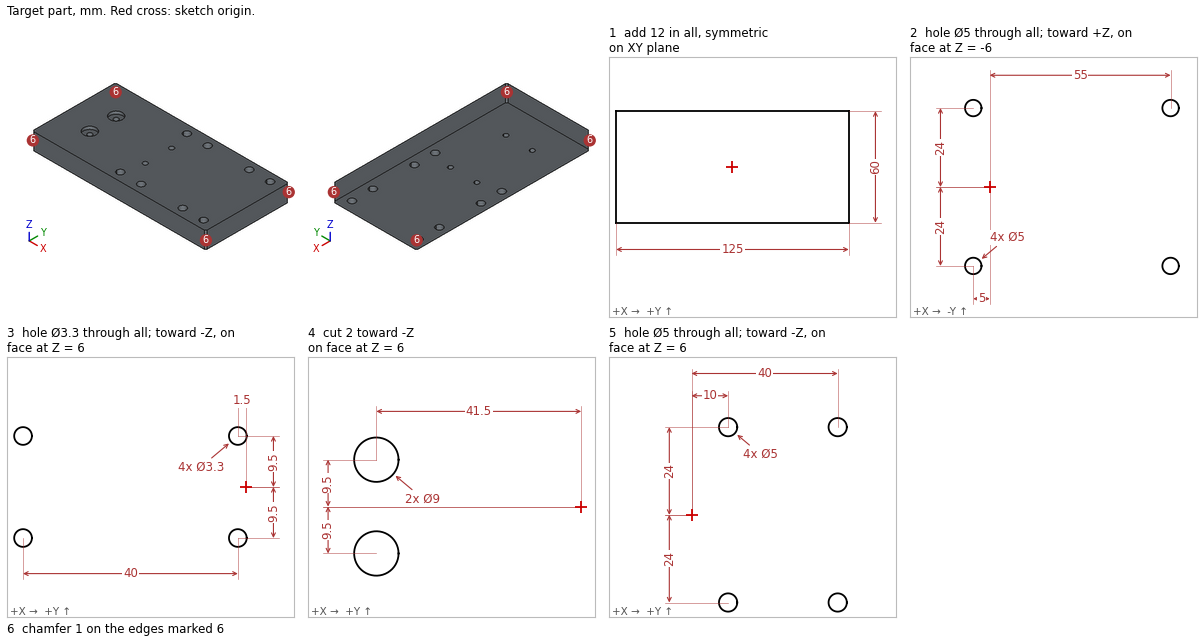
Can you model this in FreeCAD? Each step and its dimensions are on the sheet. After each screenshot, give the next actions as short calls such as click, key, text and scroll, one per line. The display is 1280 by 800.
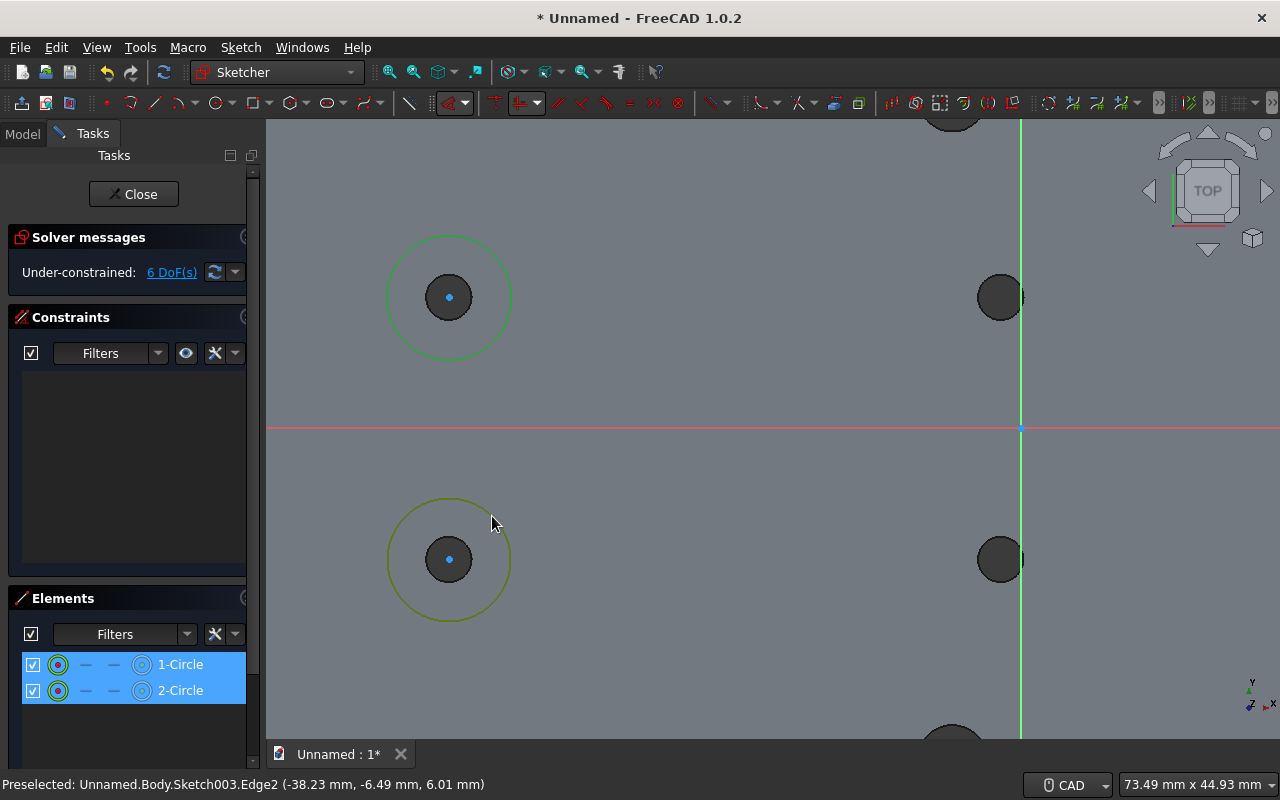
click(630, 104)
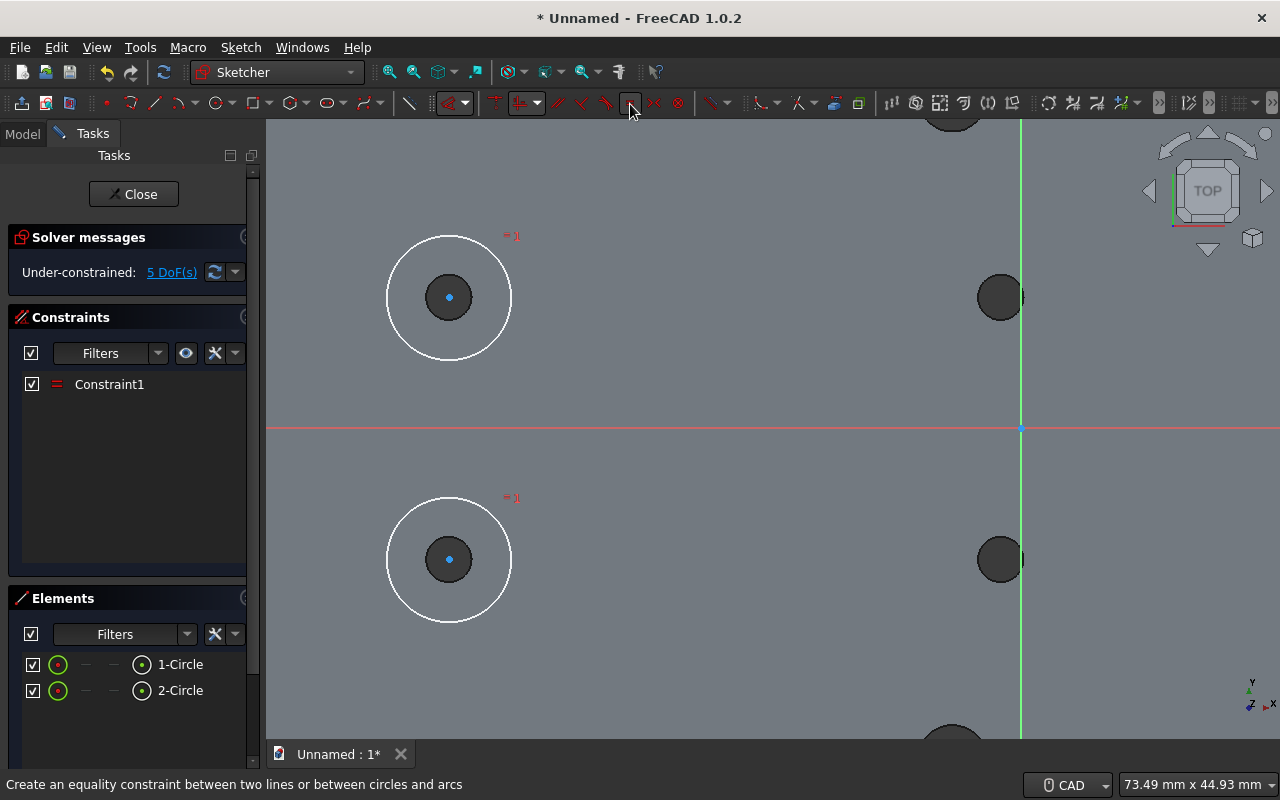
click(449, 298)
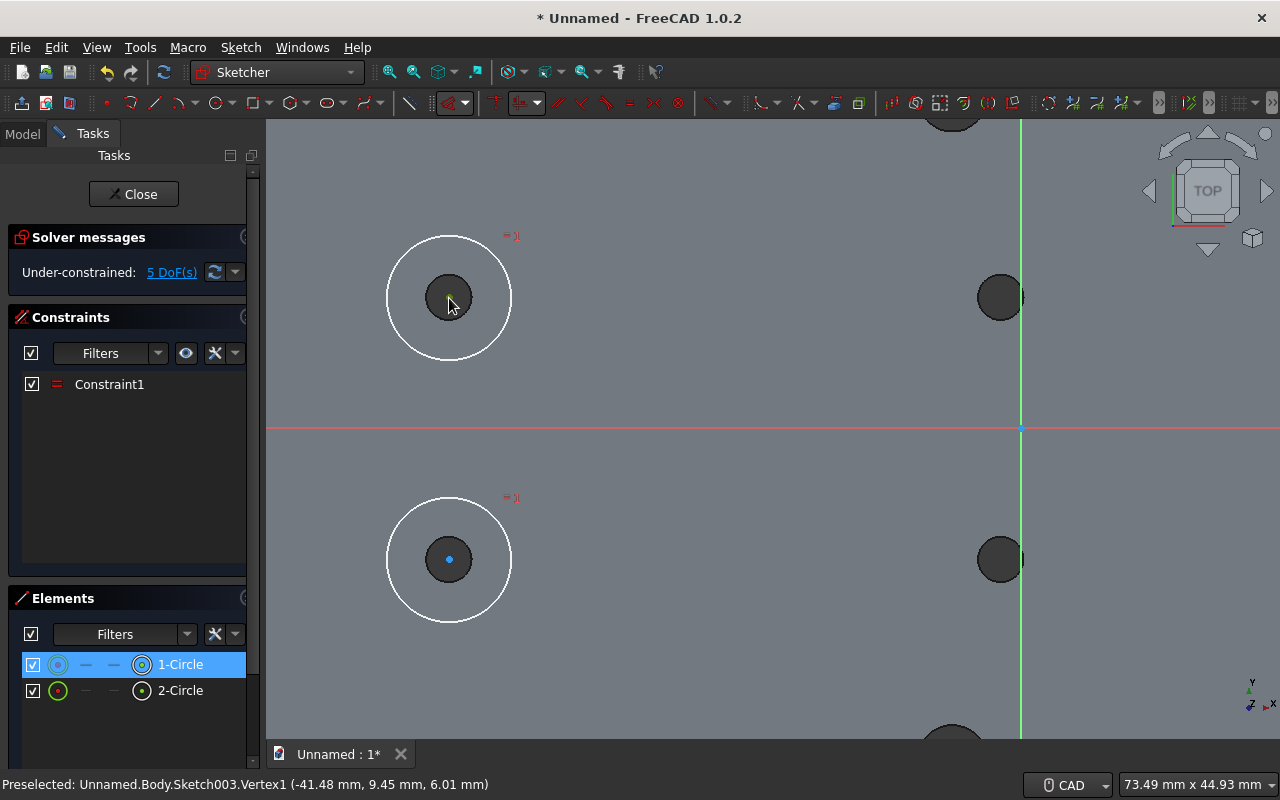
click(449, 560)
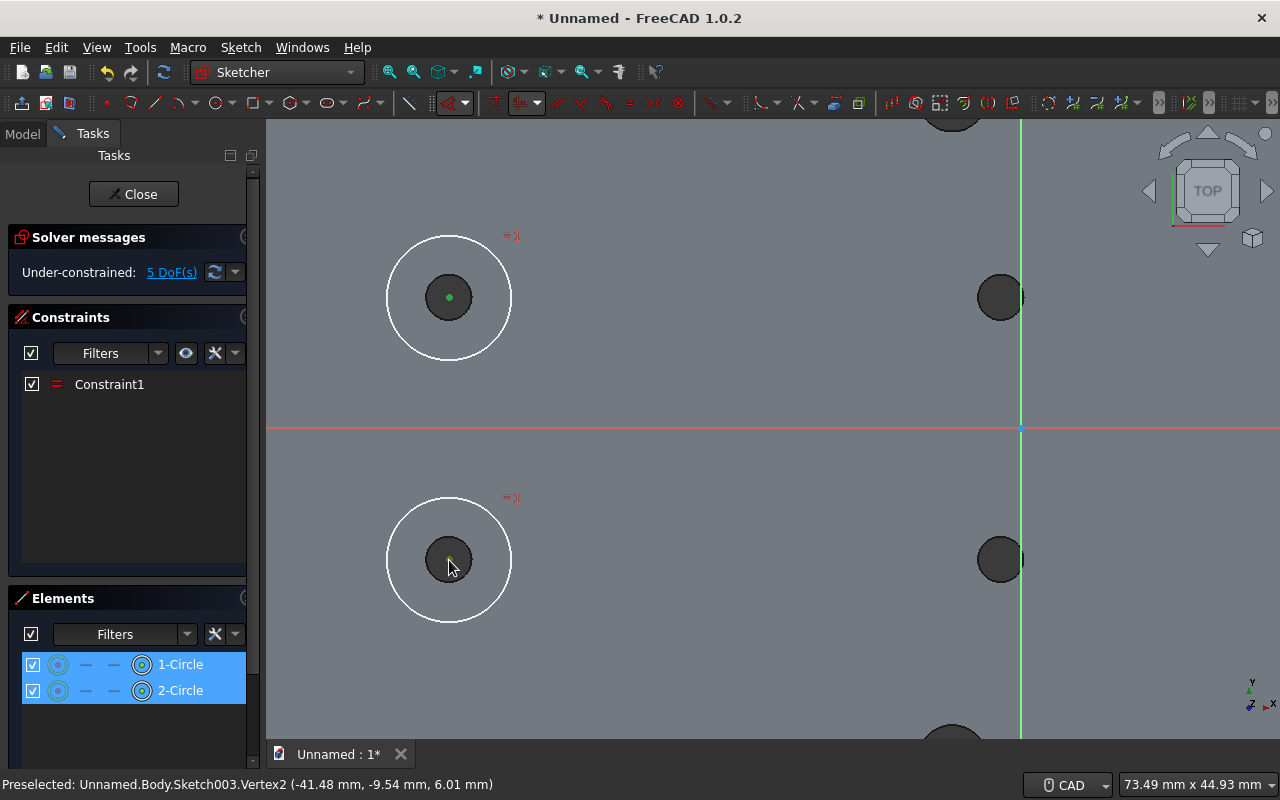
key(v)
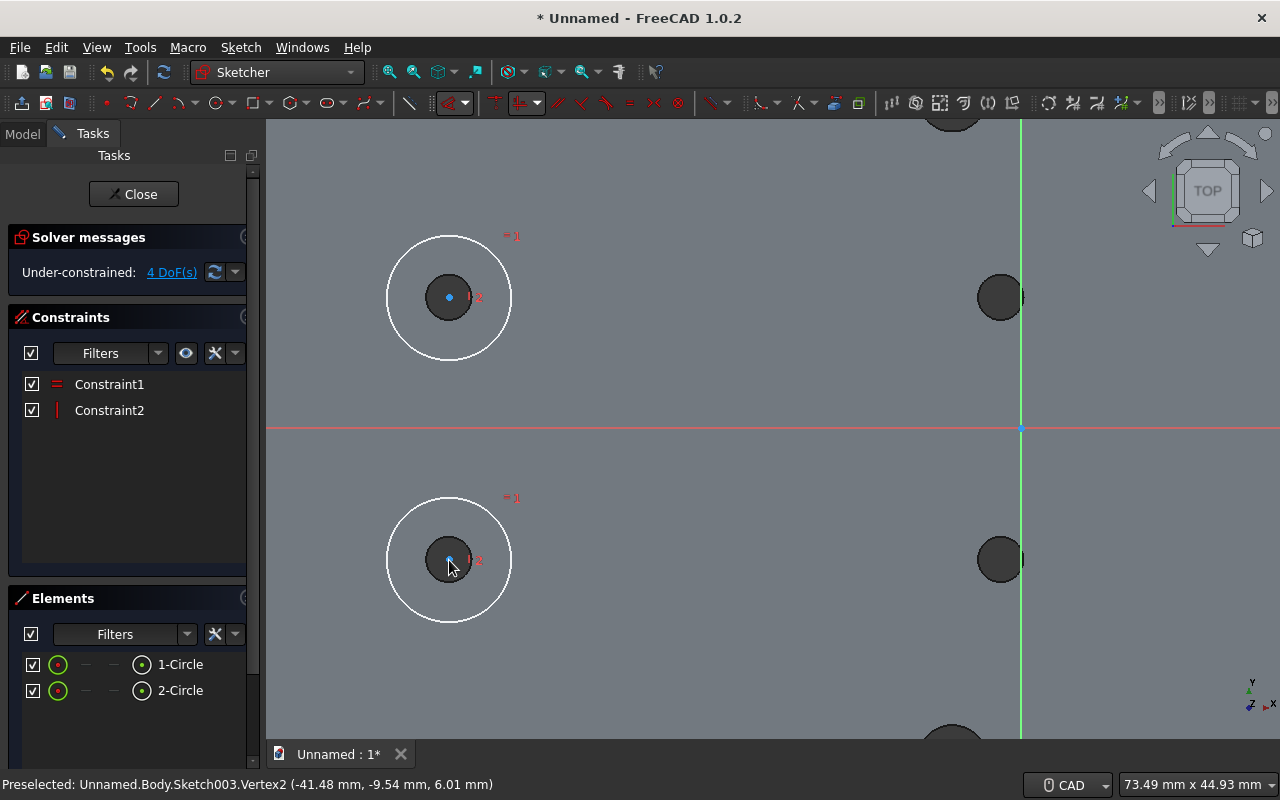
click(493, 254)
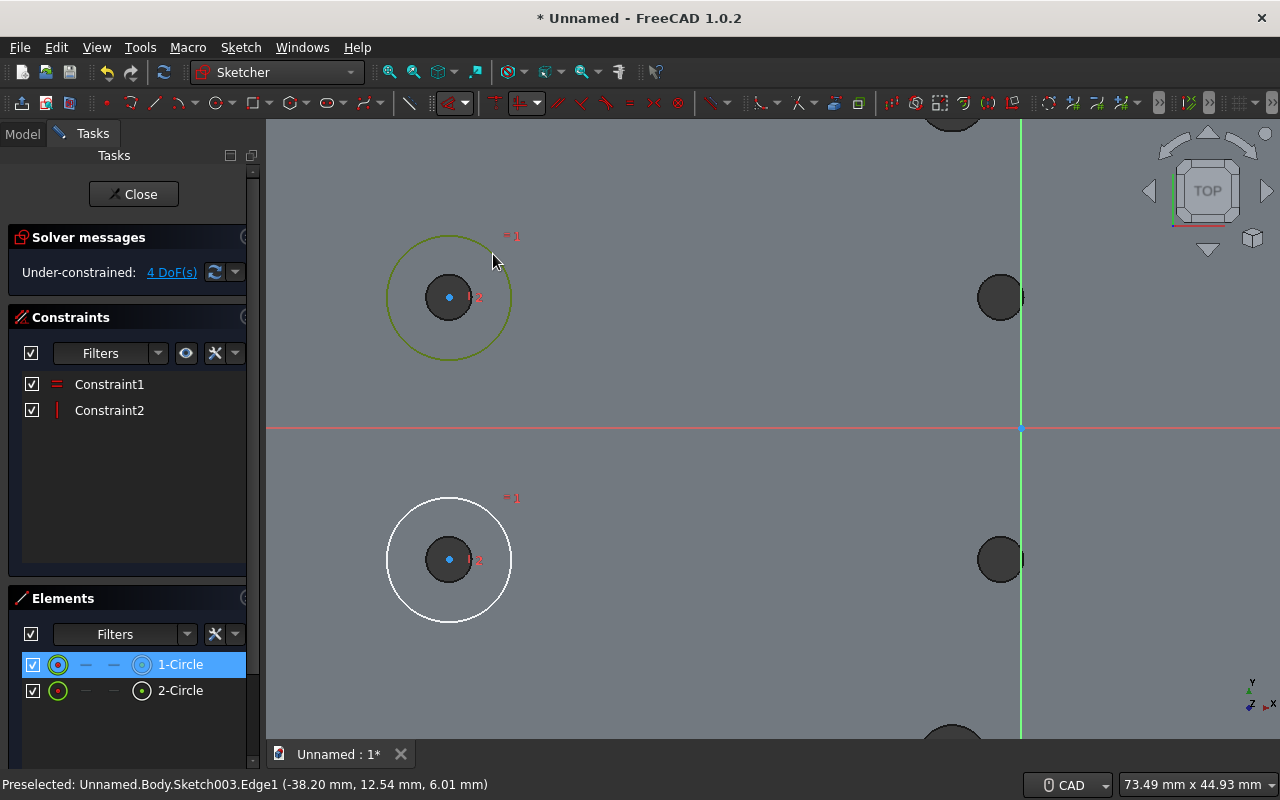
key(k)
key(o)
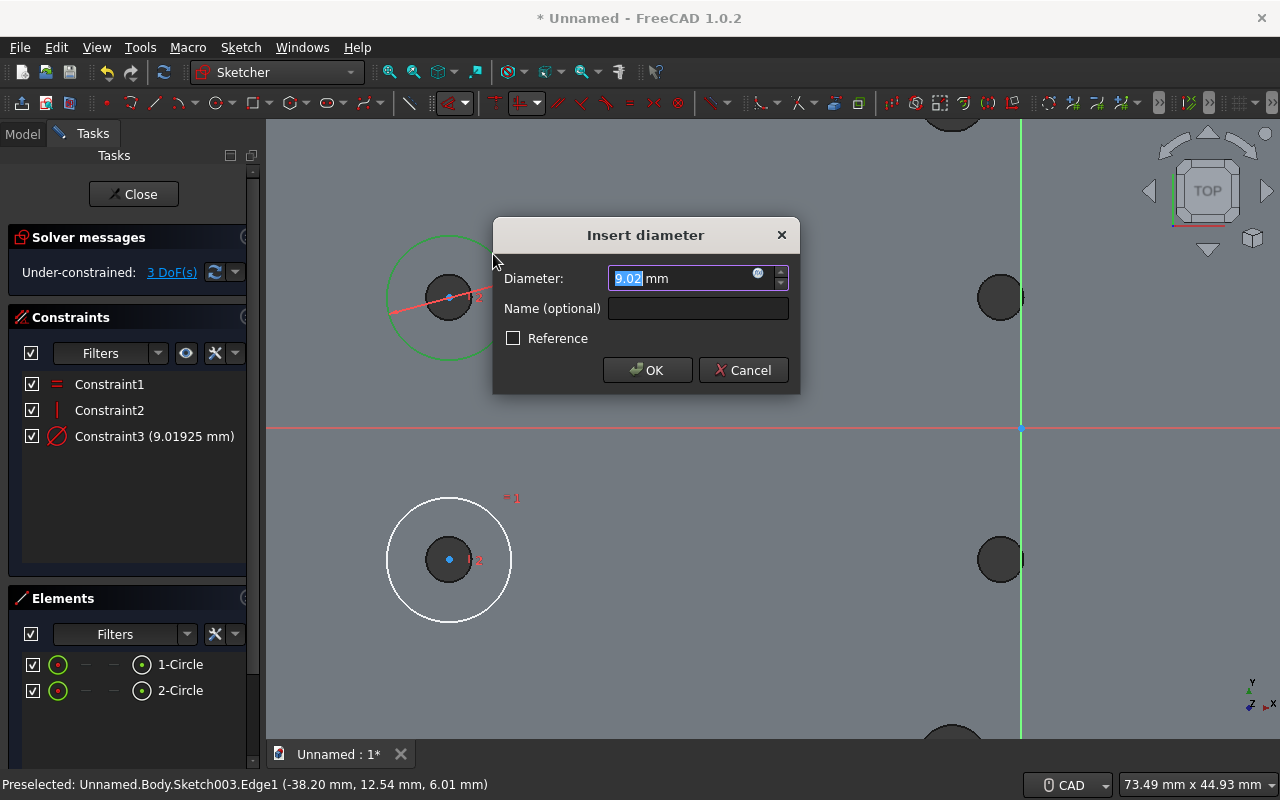
text(9)
key(Return)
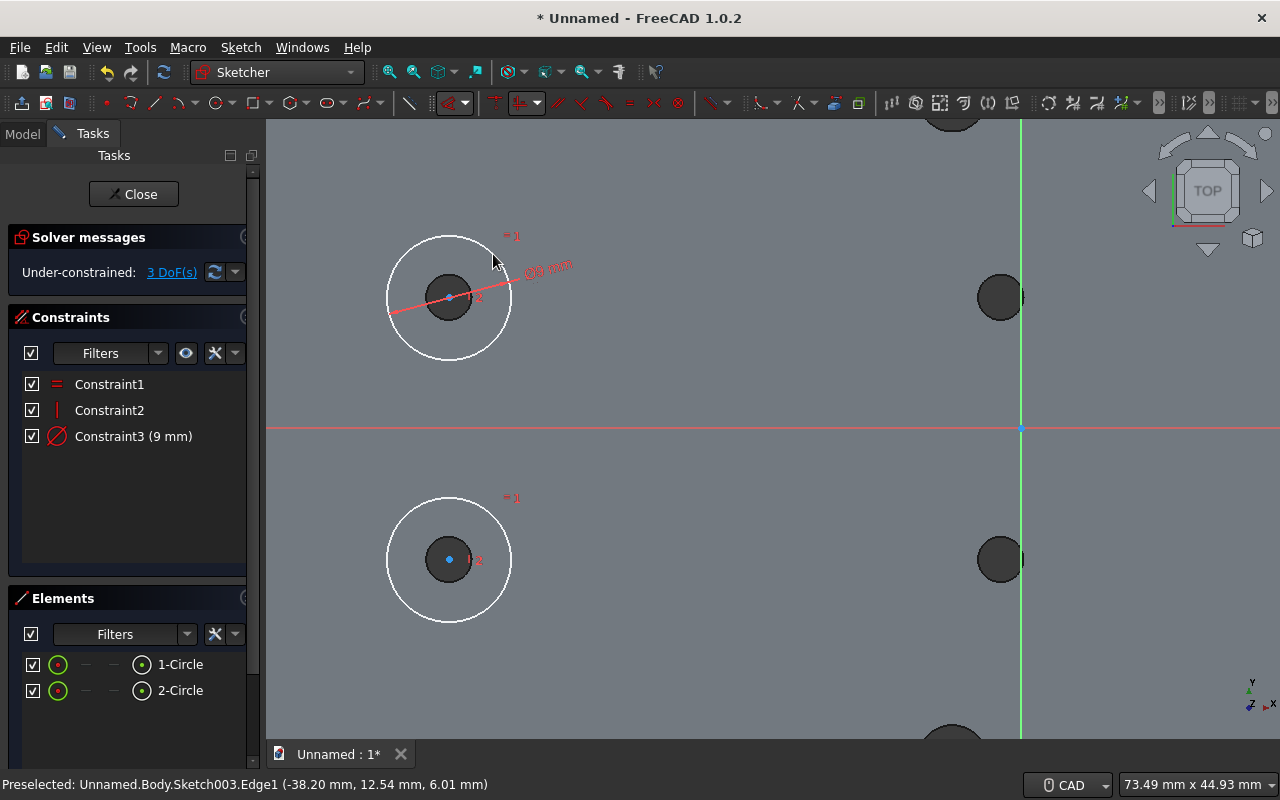
click(449, 298)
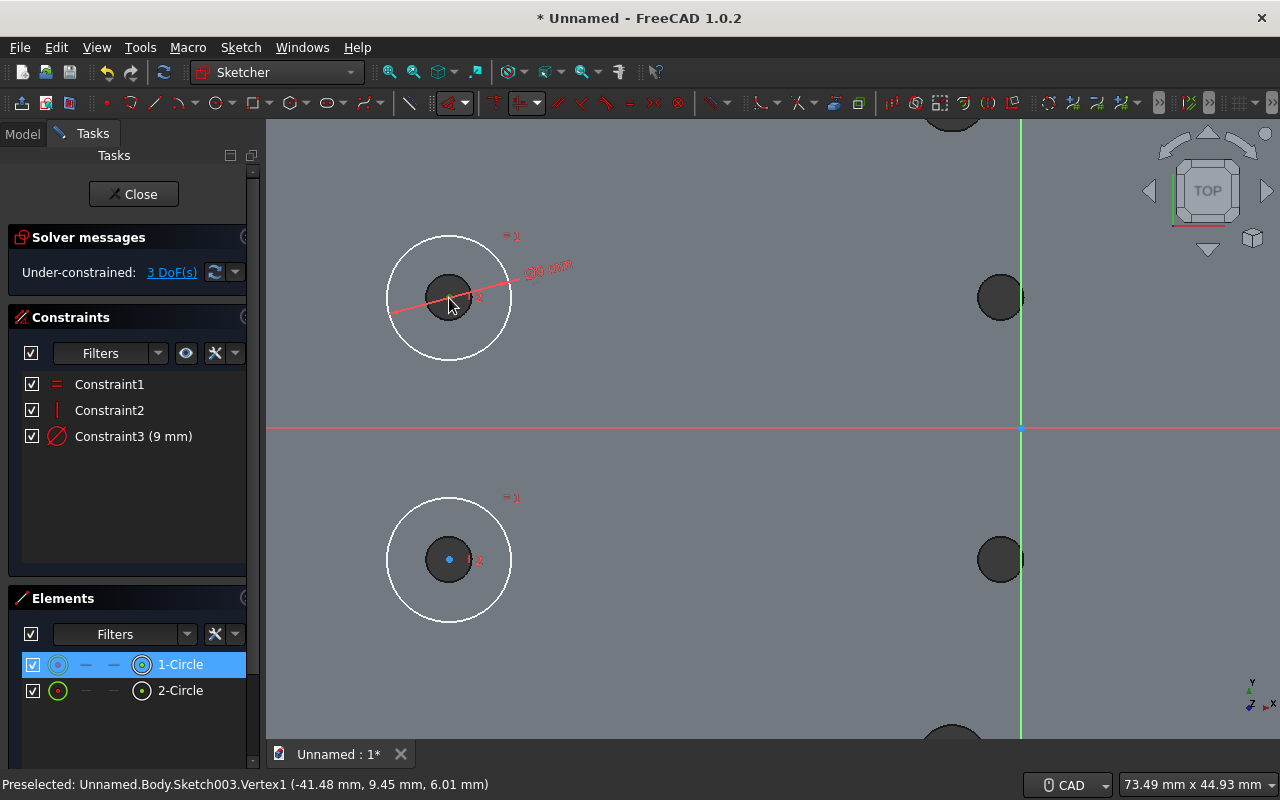
key(i)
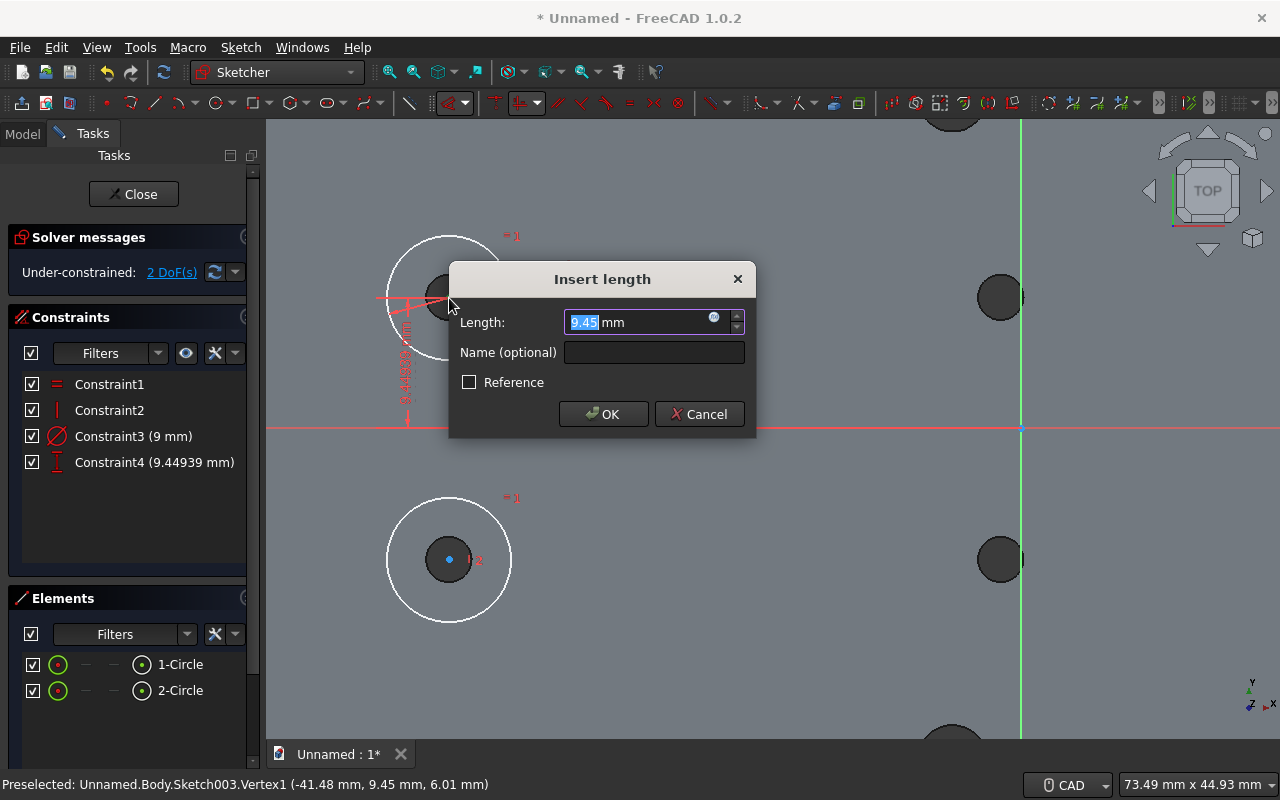
text(9.5)
key(Return)